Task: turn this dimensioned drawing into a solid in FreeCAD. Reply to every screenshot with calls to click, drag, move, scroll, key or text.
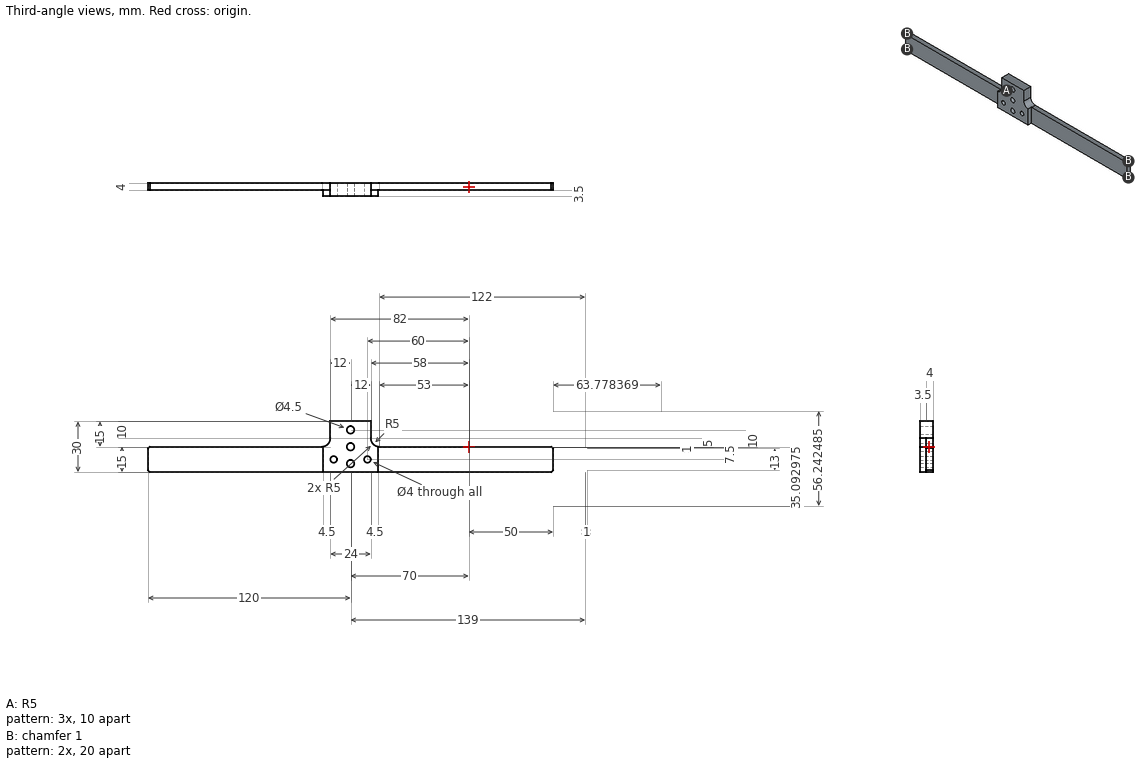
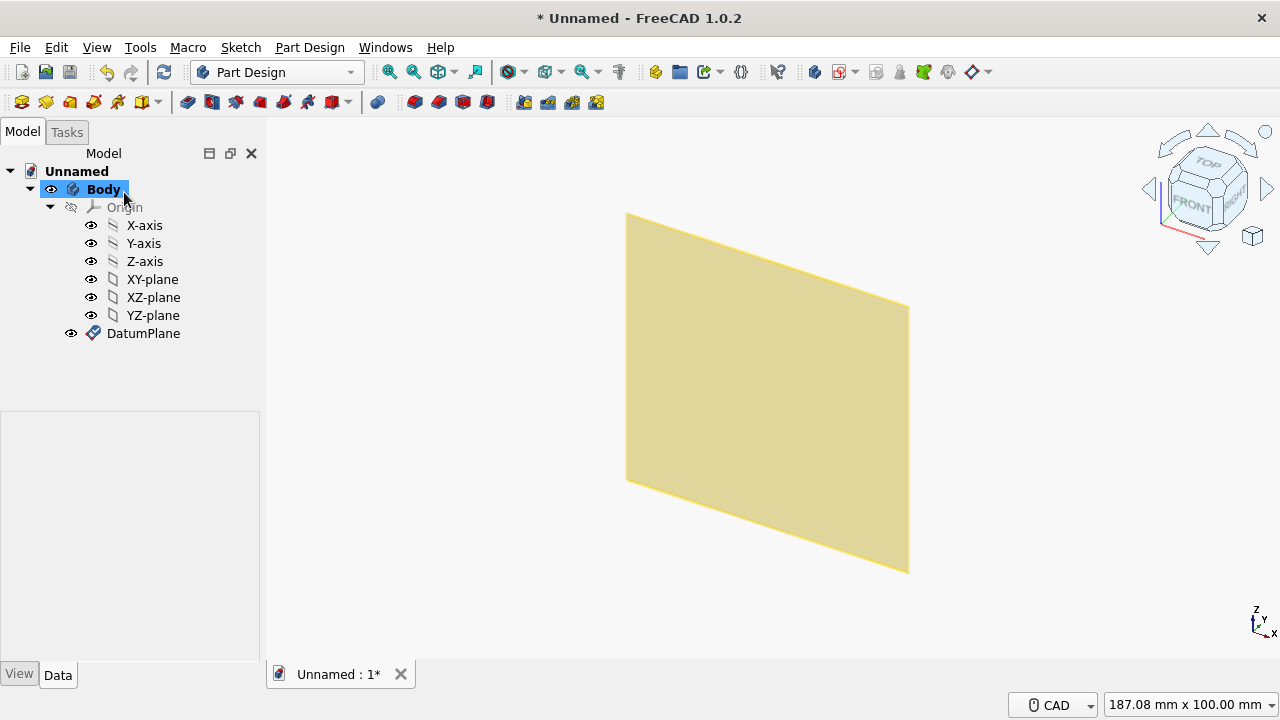
click(116, 333)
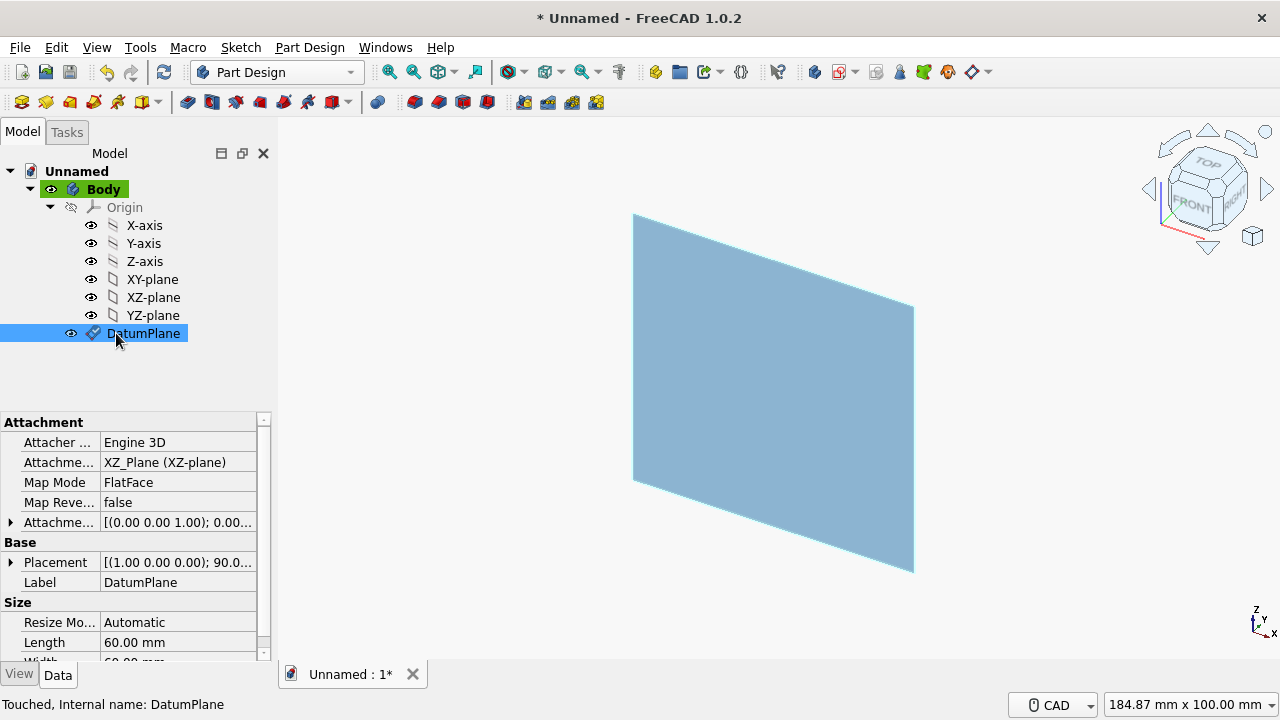
click(840, 72)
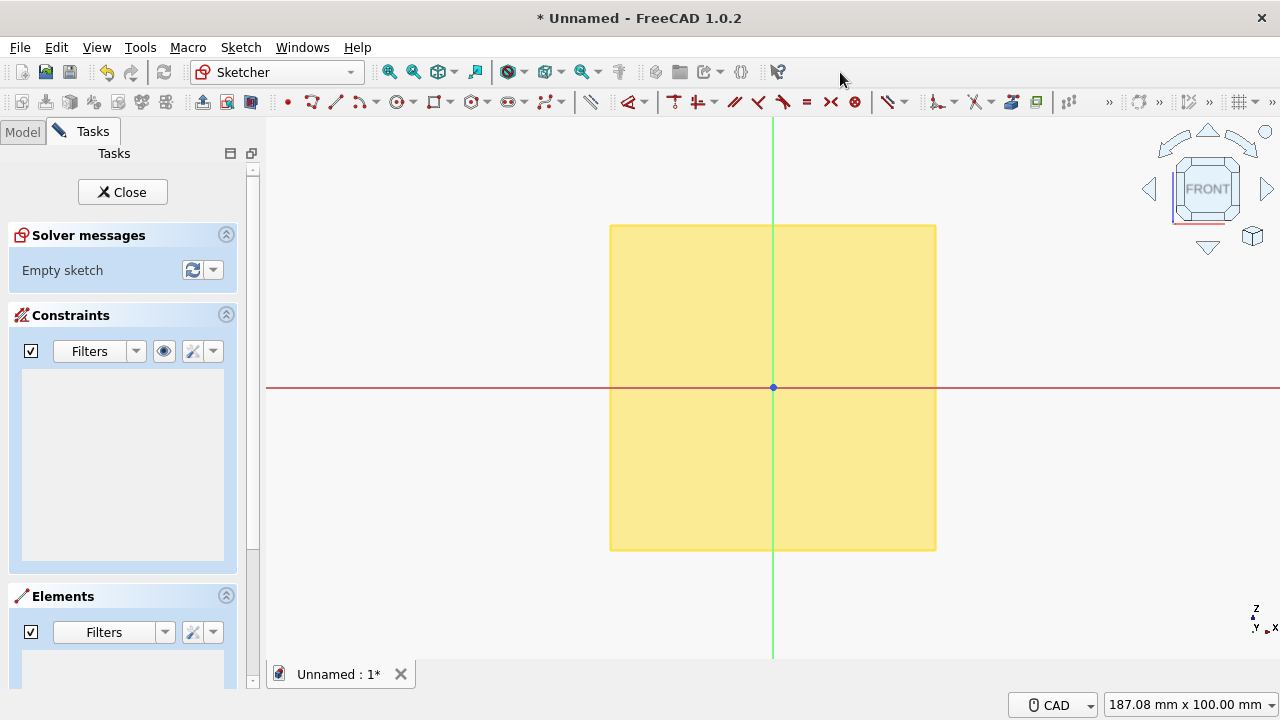
scroll(395, 388, down, 1)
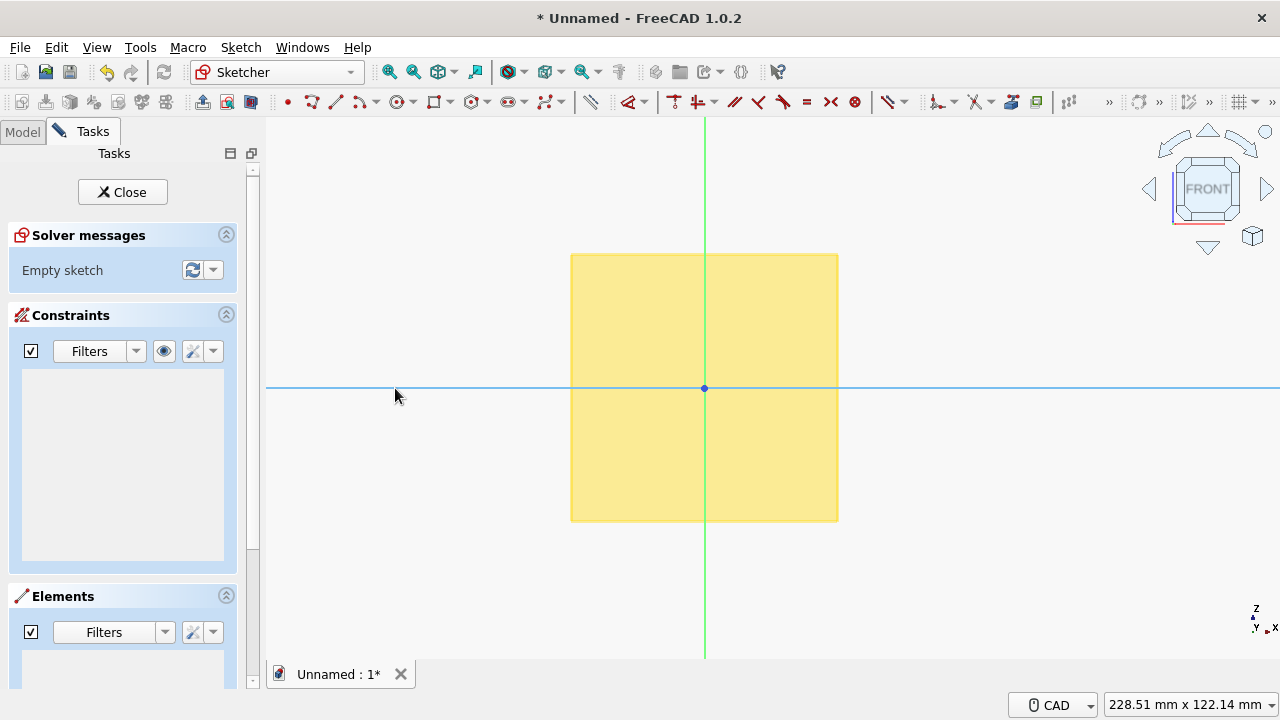
click(312, 102)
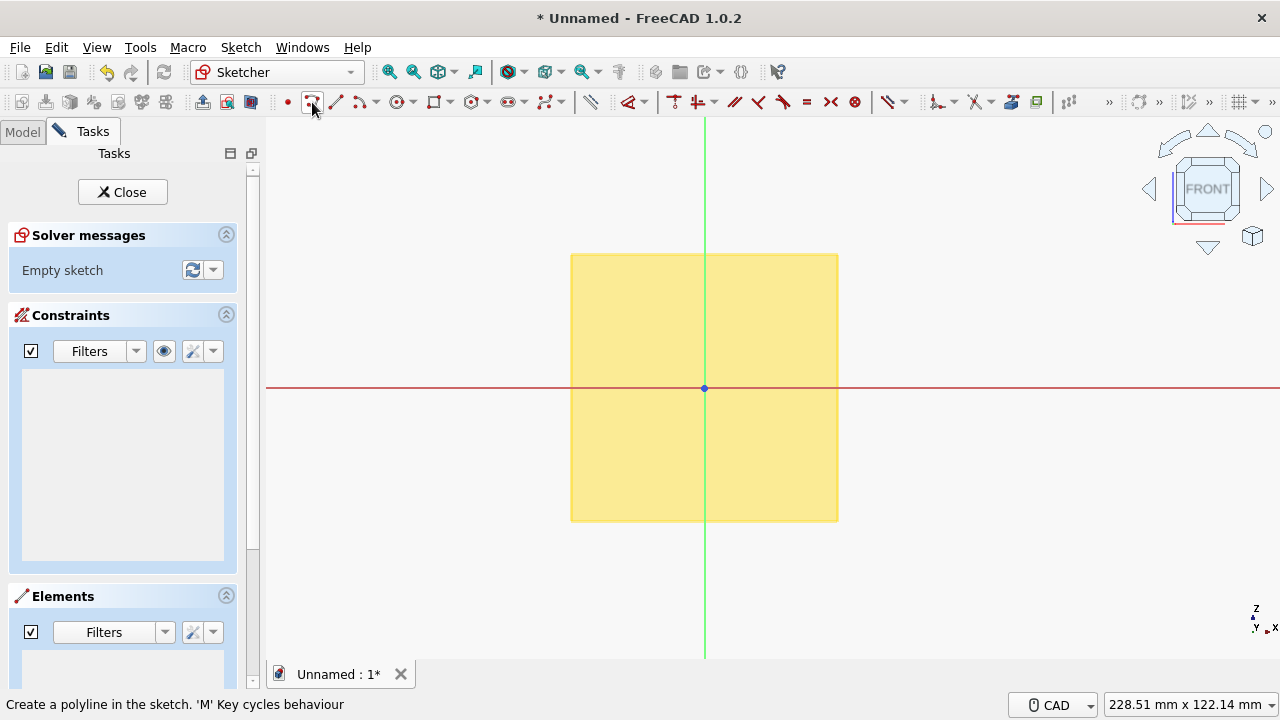
click(447, 366)
click(447, 322)
click(394, 322)
click(394, 455)
click(1011, 455)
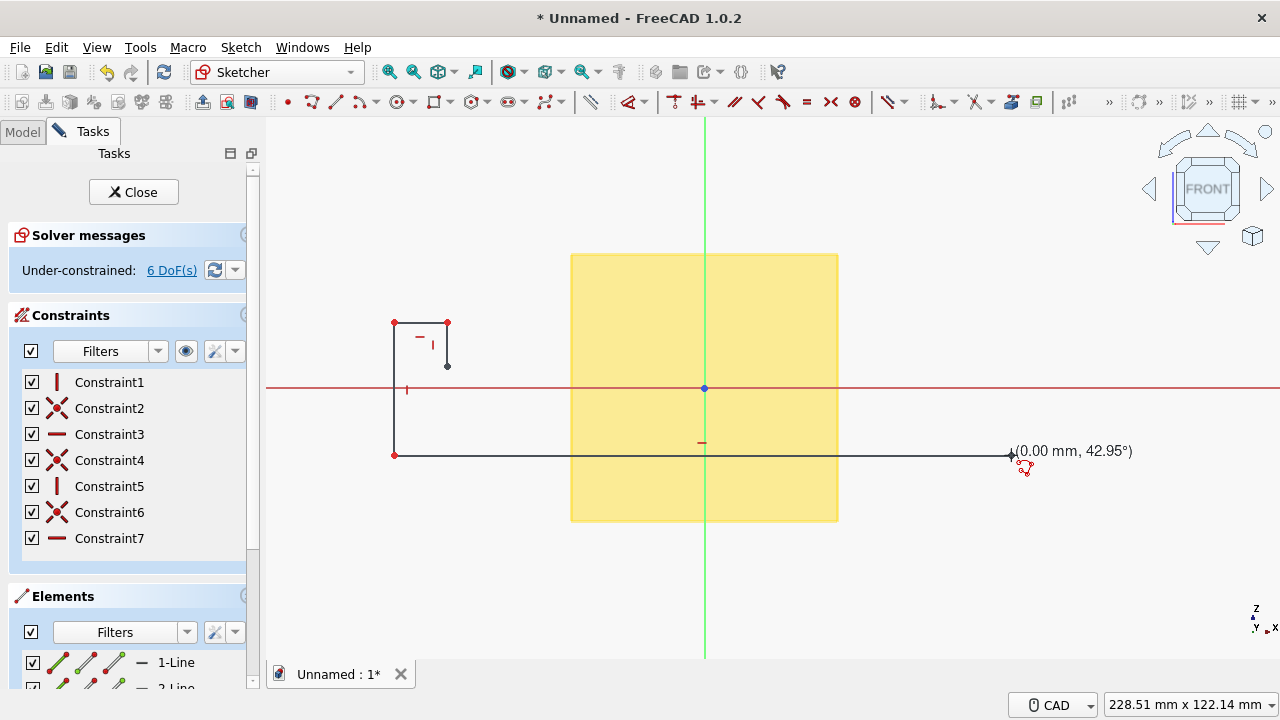
scroll(1015, 450, up, 5)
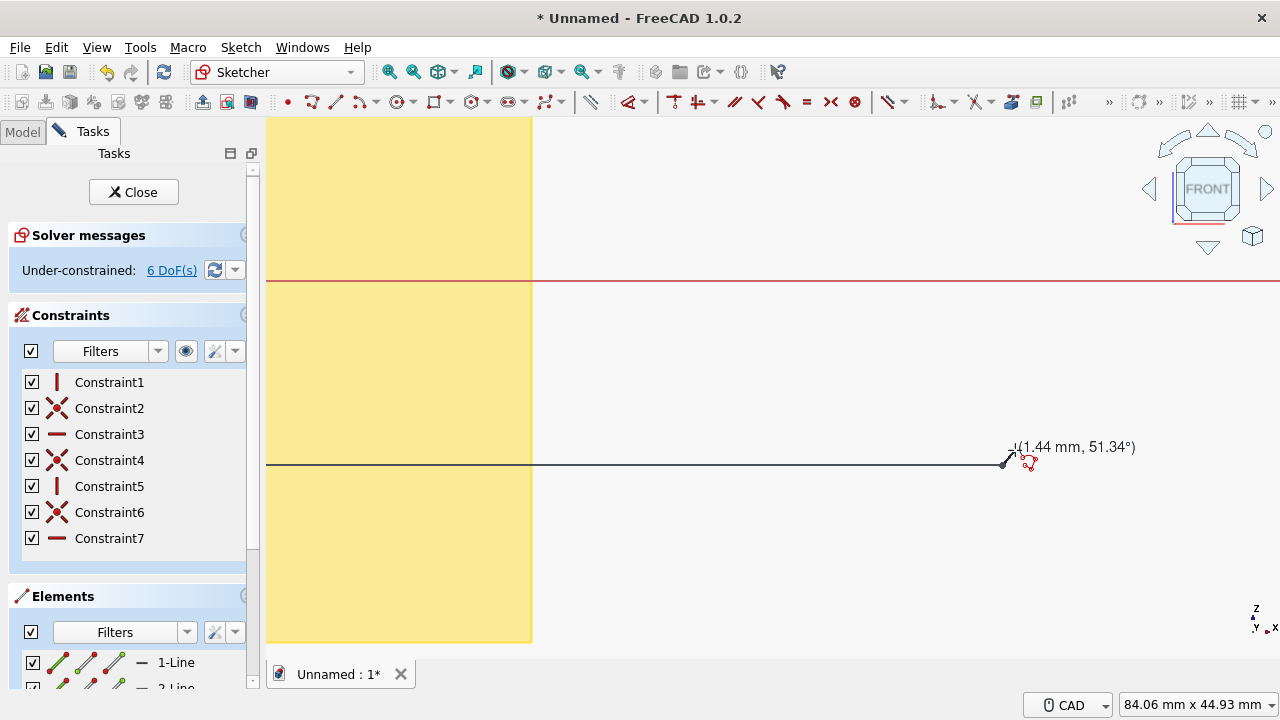
click(1014, 450)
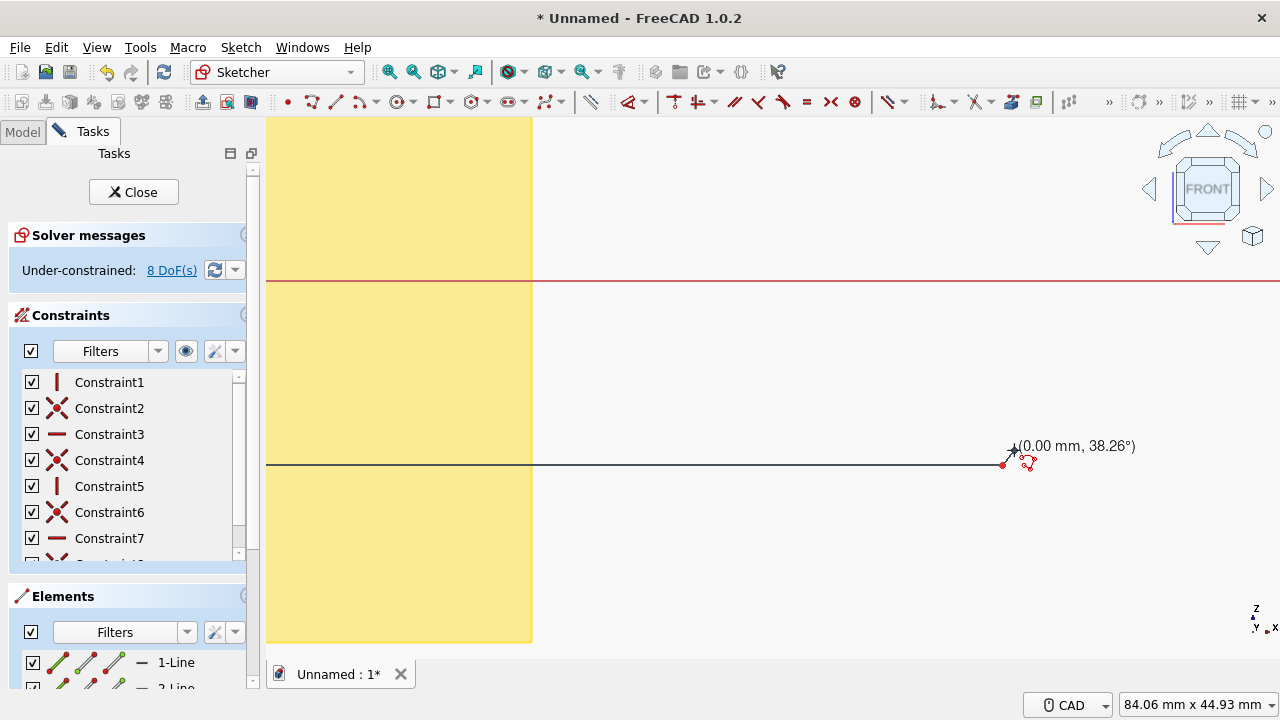
scroll(1014, 293, up, 2)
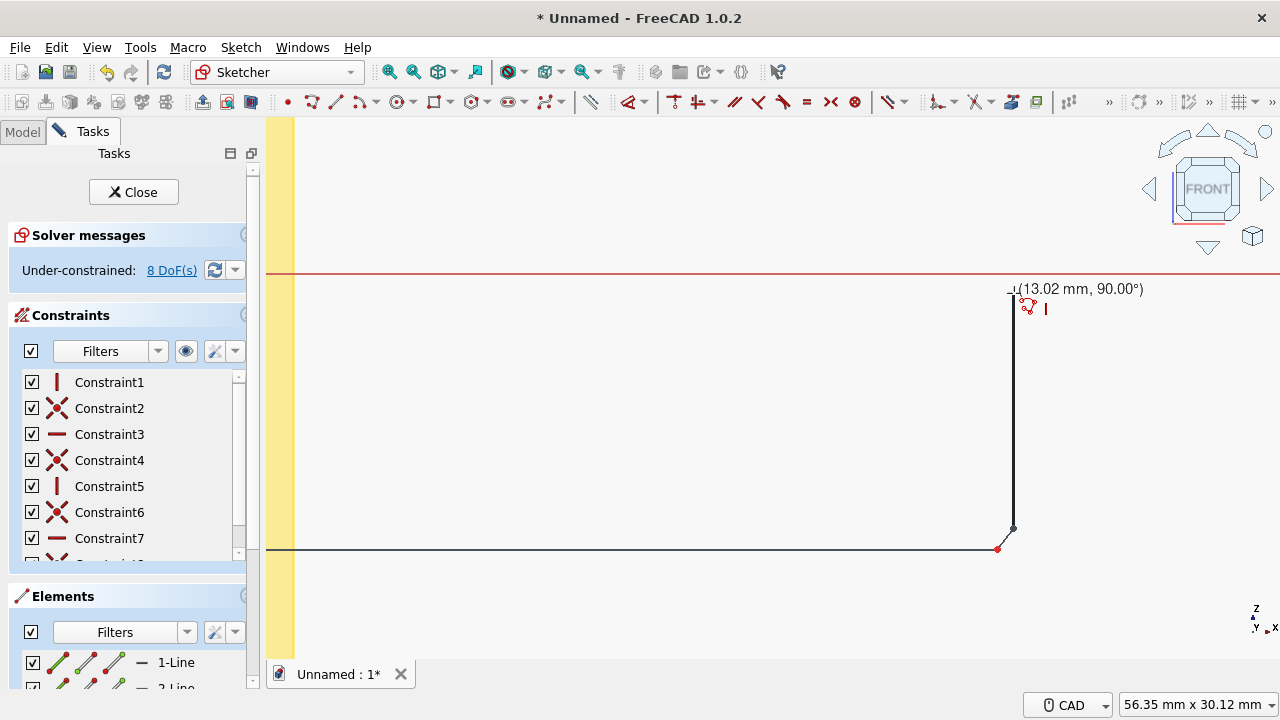
click(1014, 292)
click(996, 274)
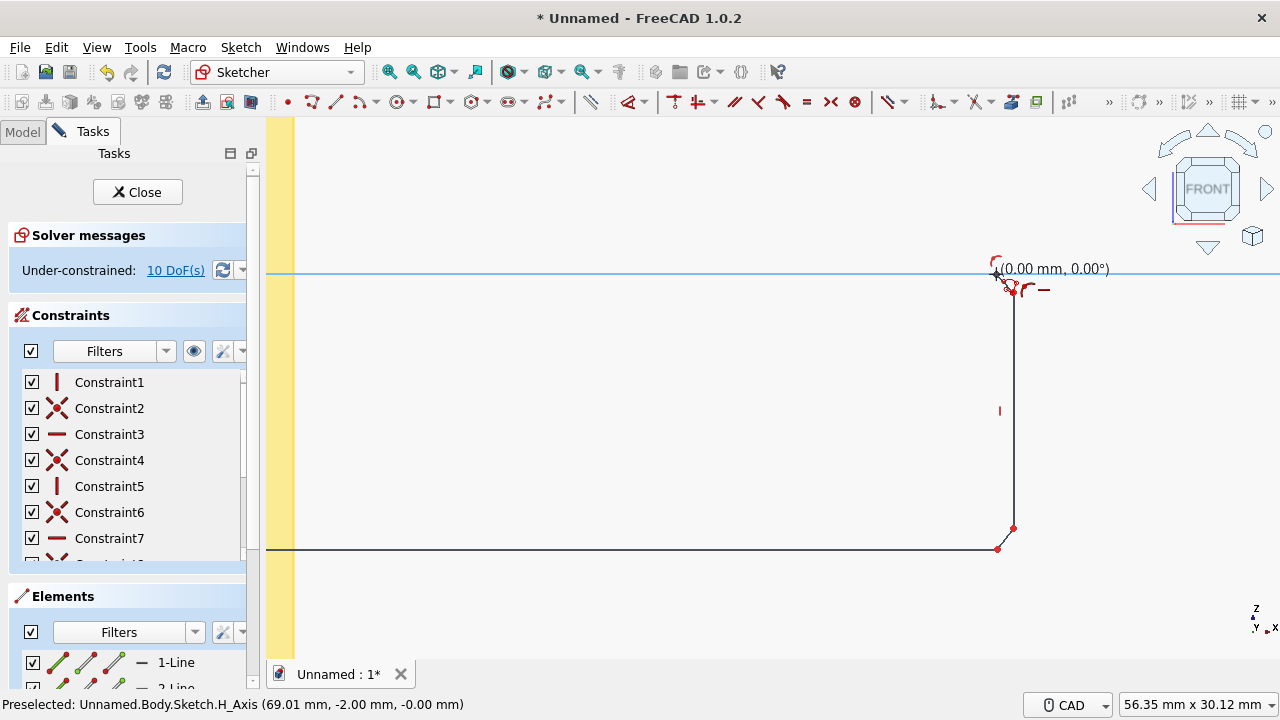
scroll(1016, 425, down, 7)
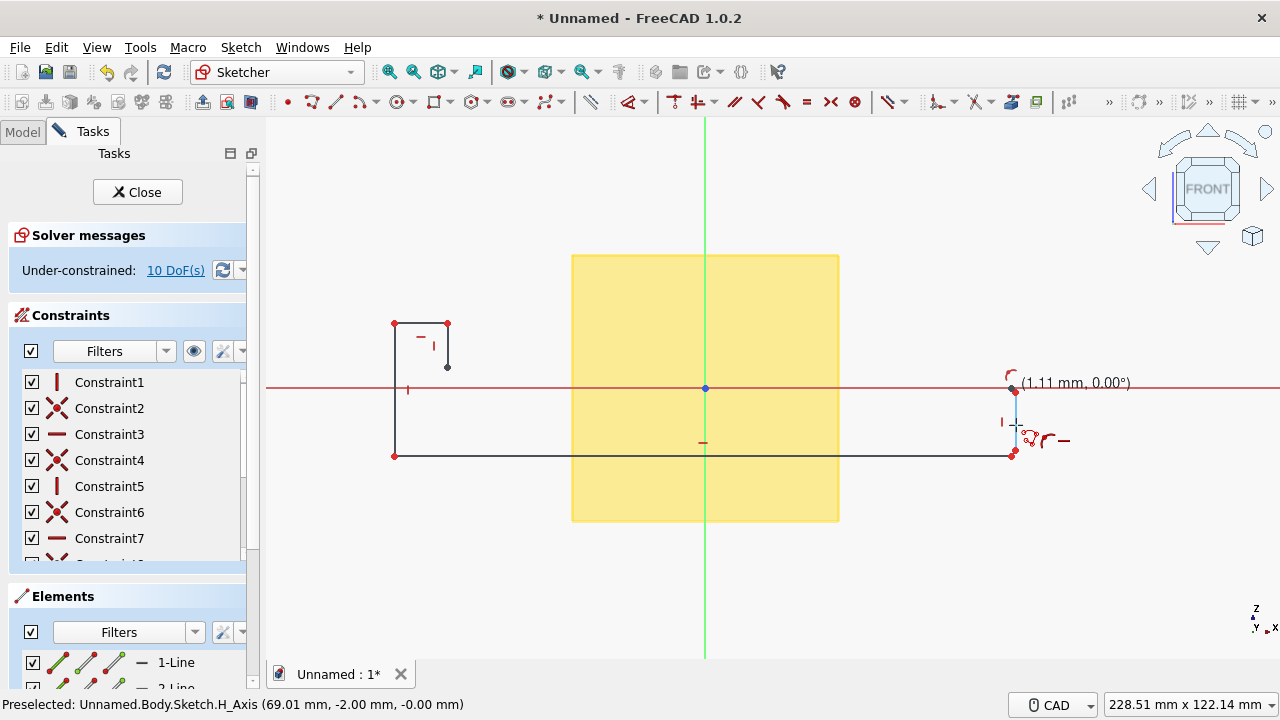
click(470, 379)
right_click(470, 379)